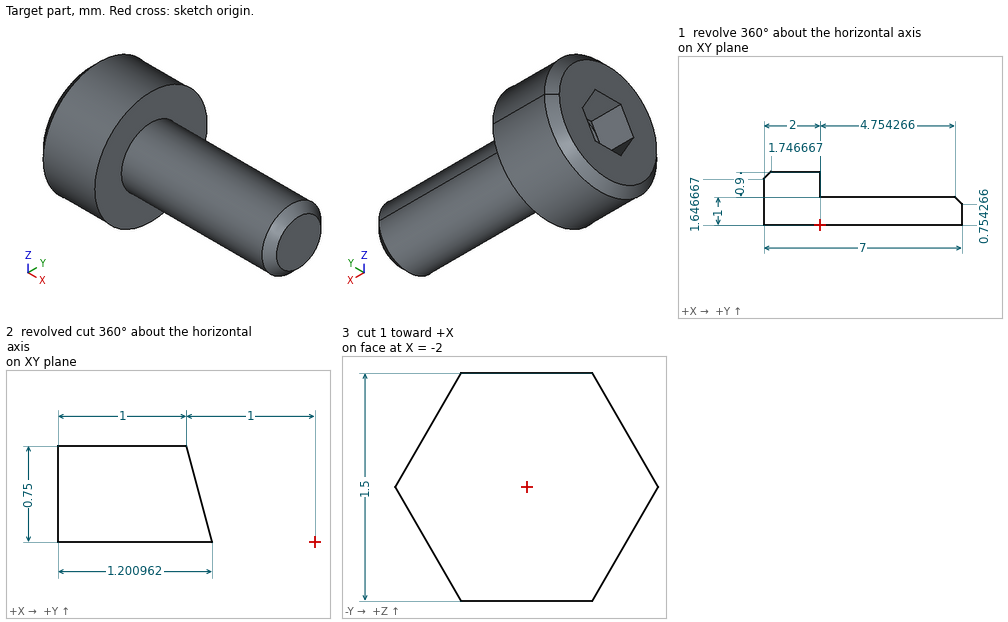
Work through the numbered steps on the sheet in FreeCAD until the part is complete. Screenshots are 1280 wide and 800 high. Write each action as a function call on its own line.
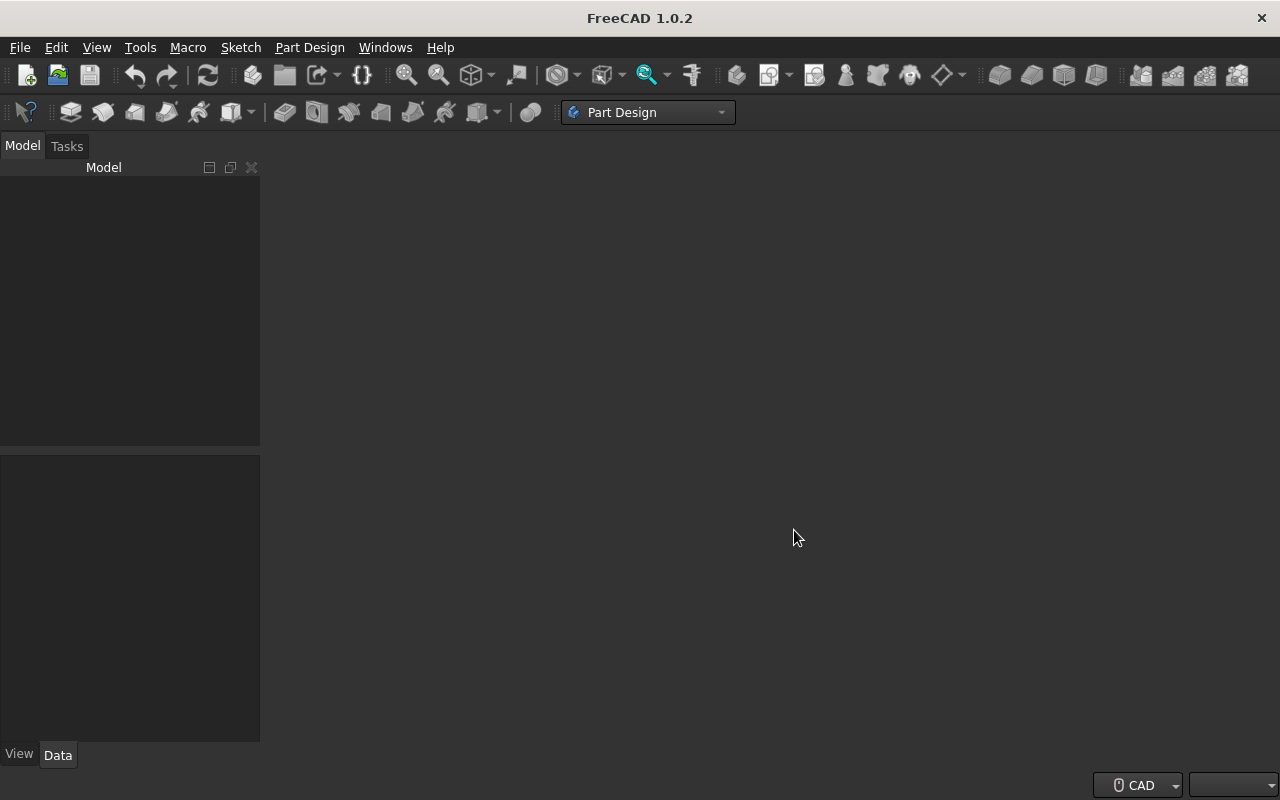
click(26, 76)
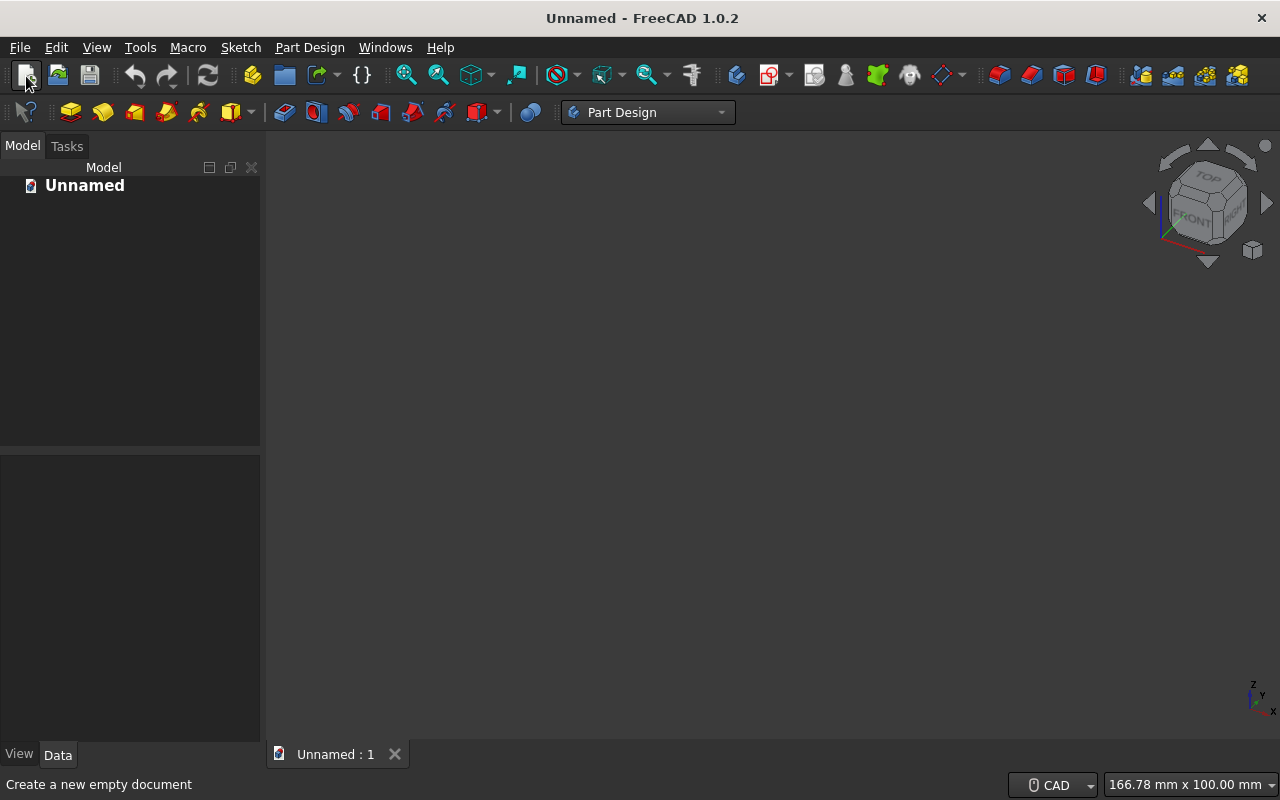
click(770, 76)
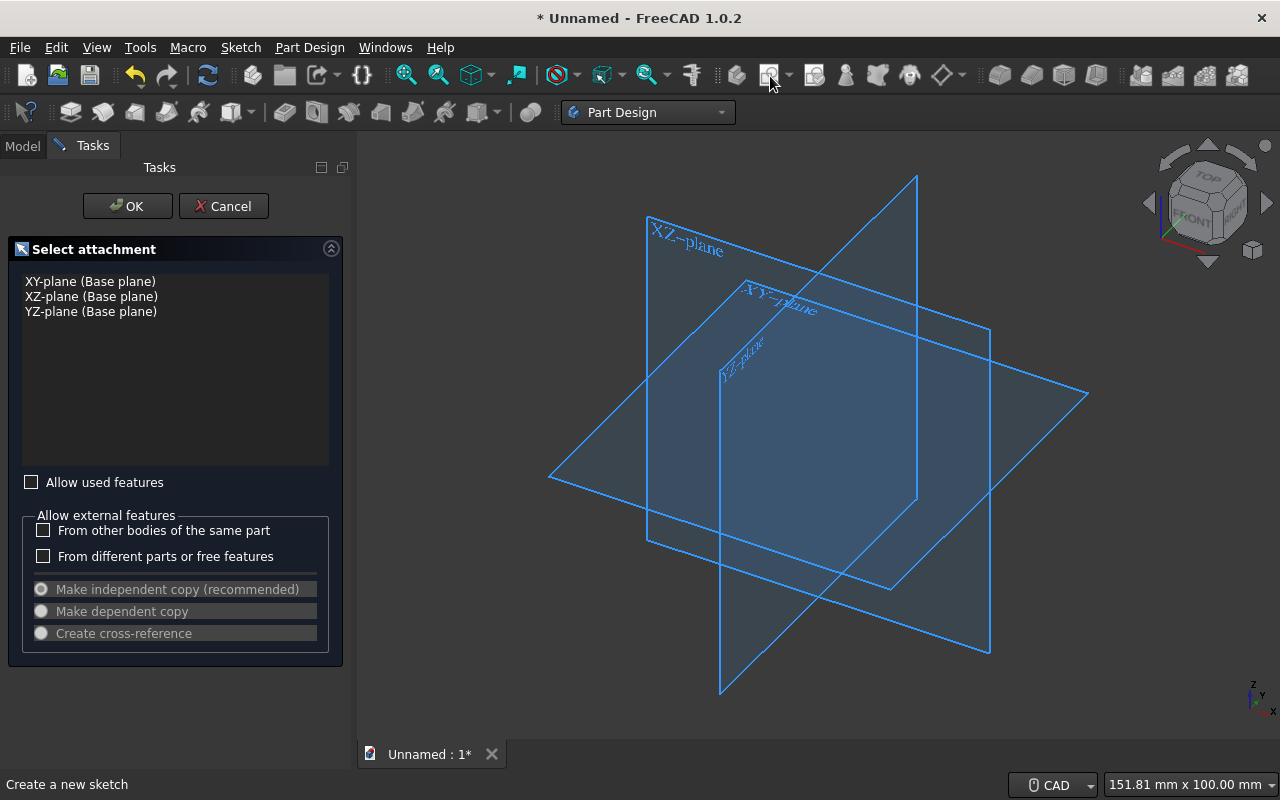
click(82, 282)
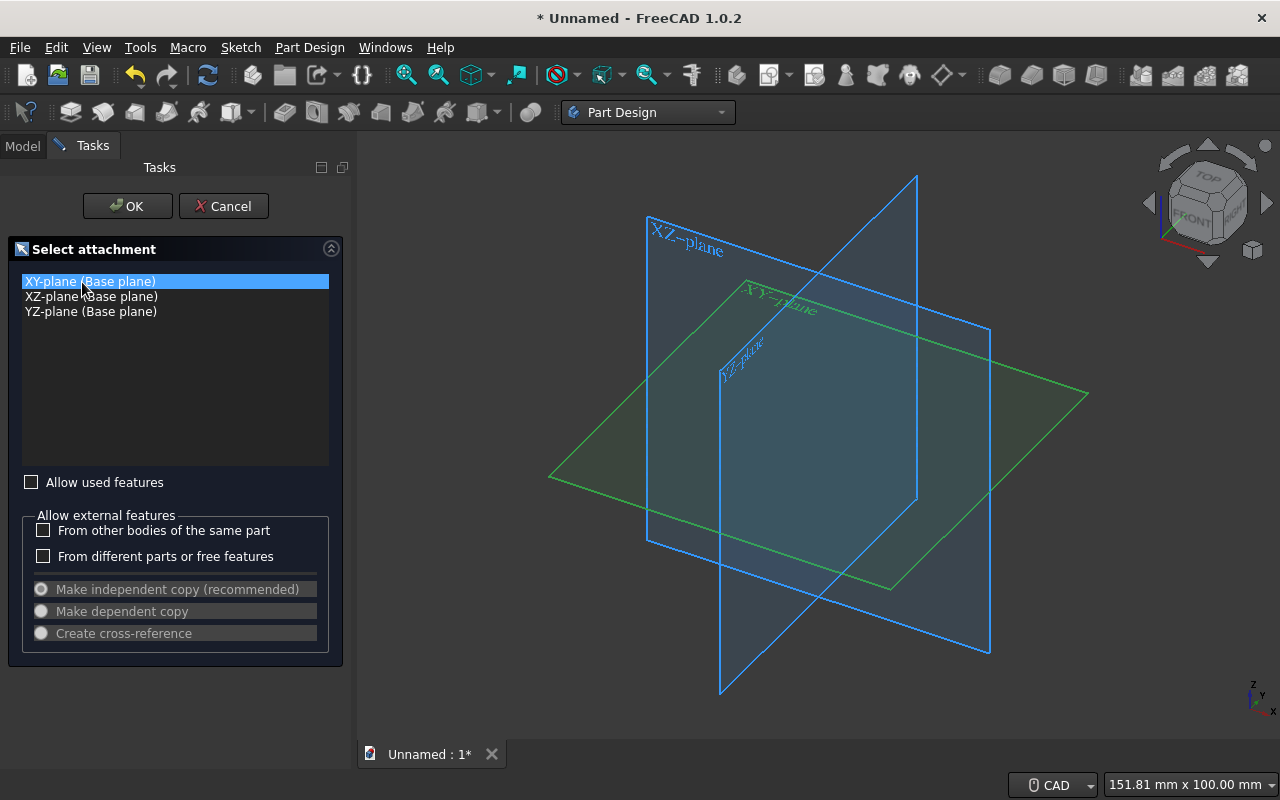
click(128, 206)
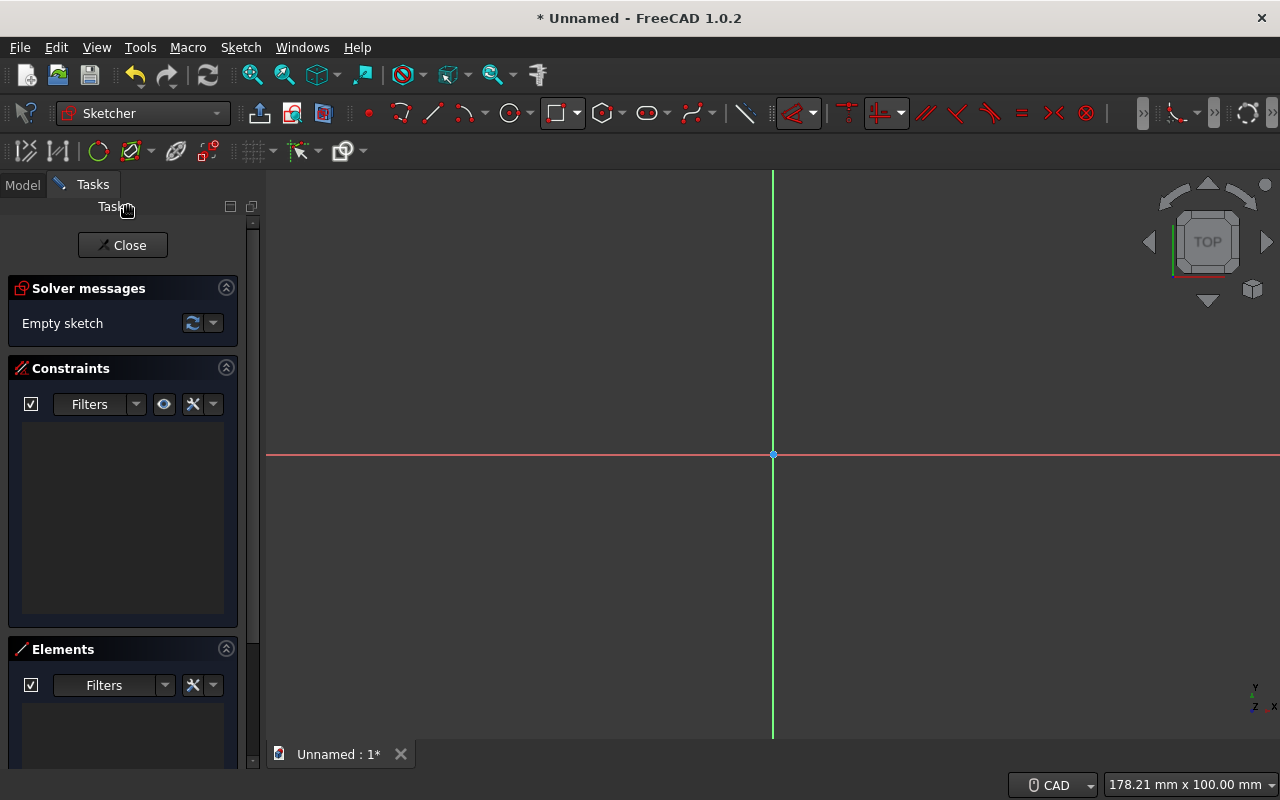
scroll(788, 449, up, 13)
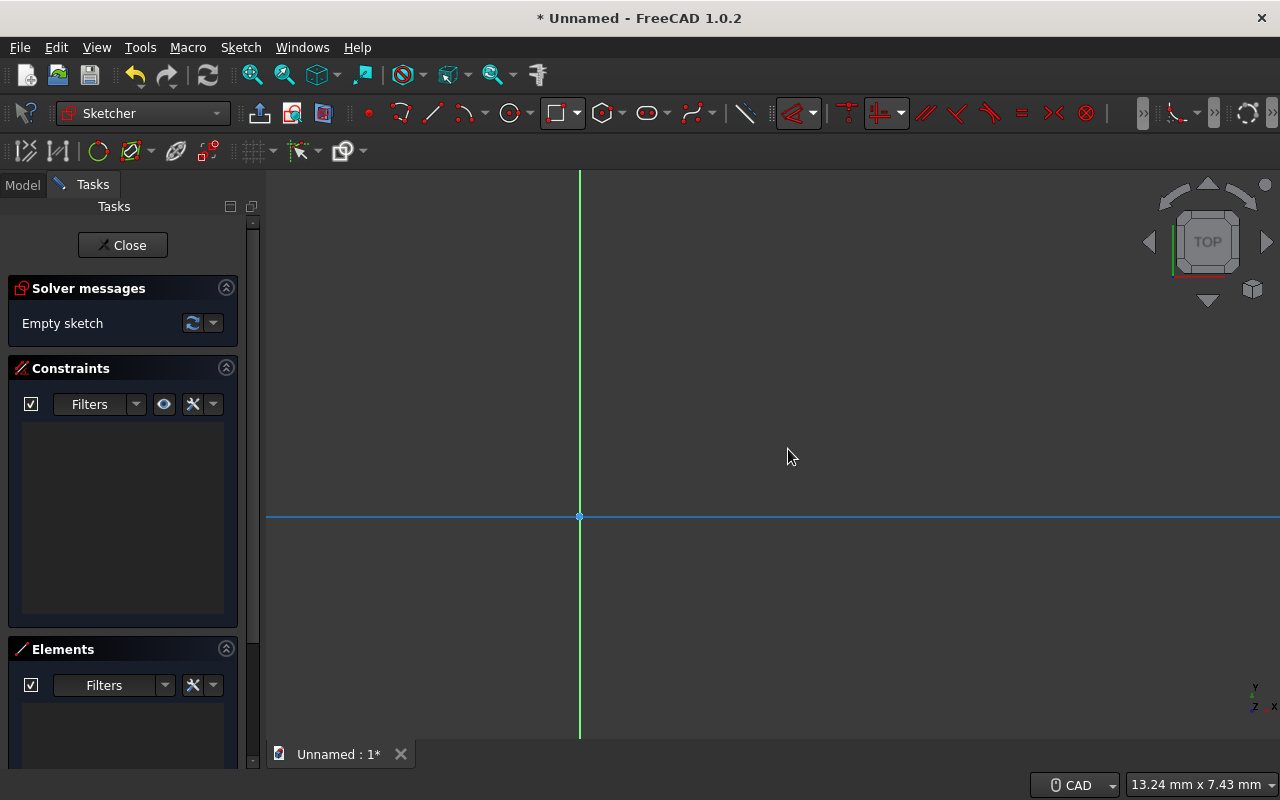
click(402, 114)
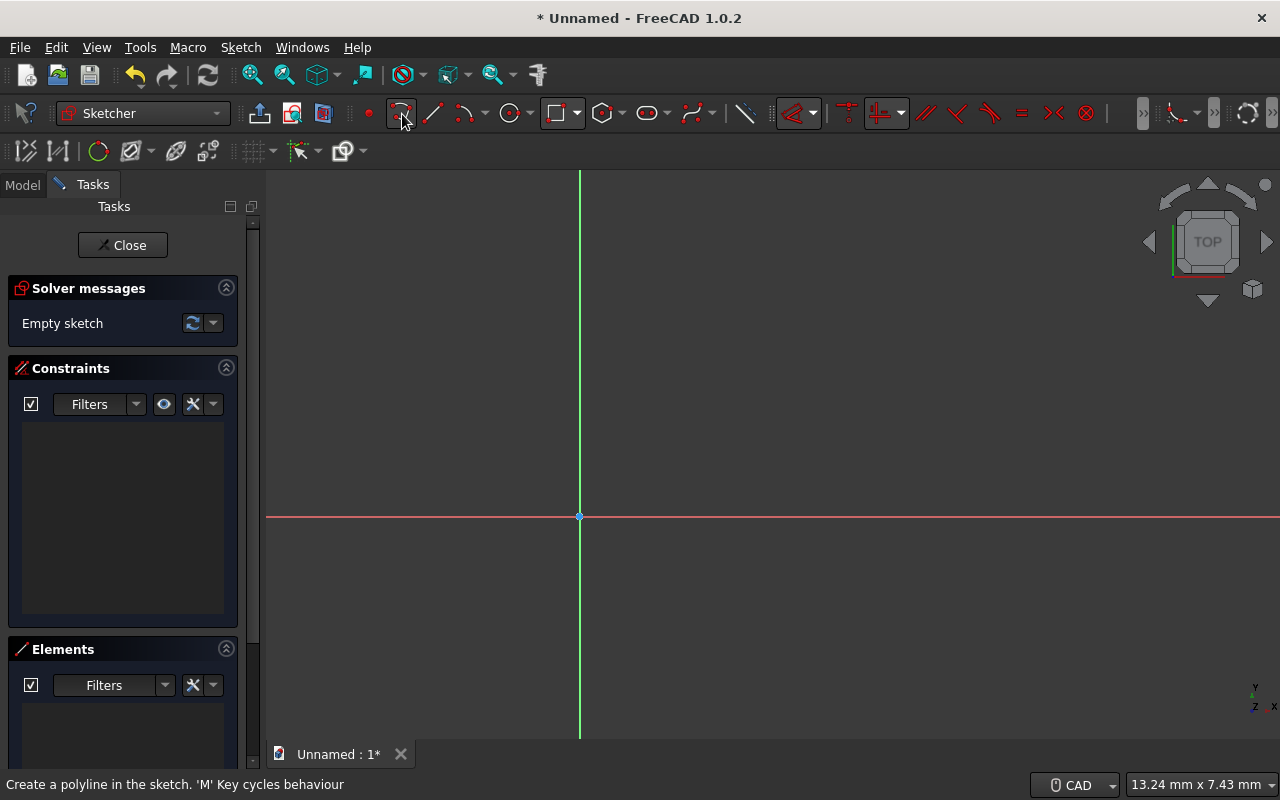
click(580, 440)
click(589, 371)
click(446, 371)
click(426, 391)
click(426, 517)
click(963, 508)
click(963, 459)
click(944, 440)
click(580, 441)
key(Escape)
key(Escape)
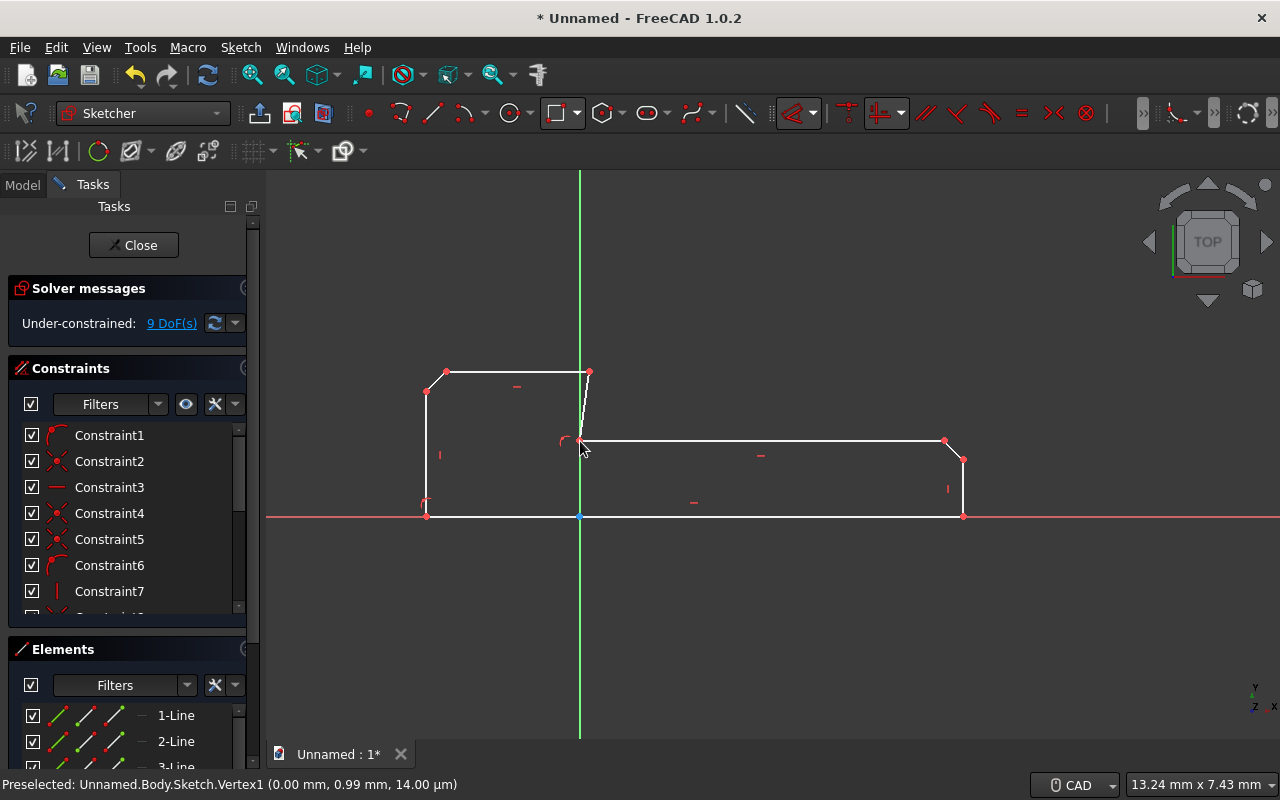
click(582, 420)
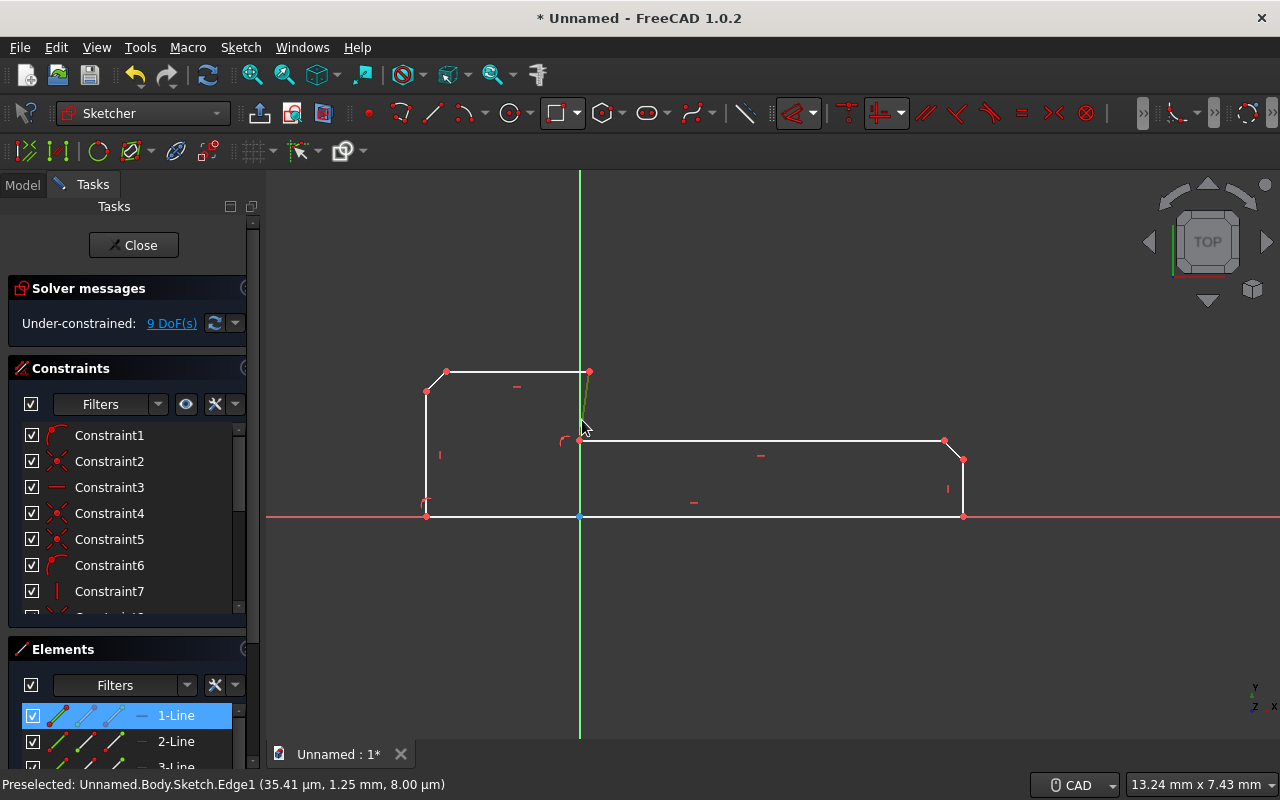
key(v)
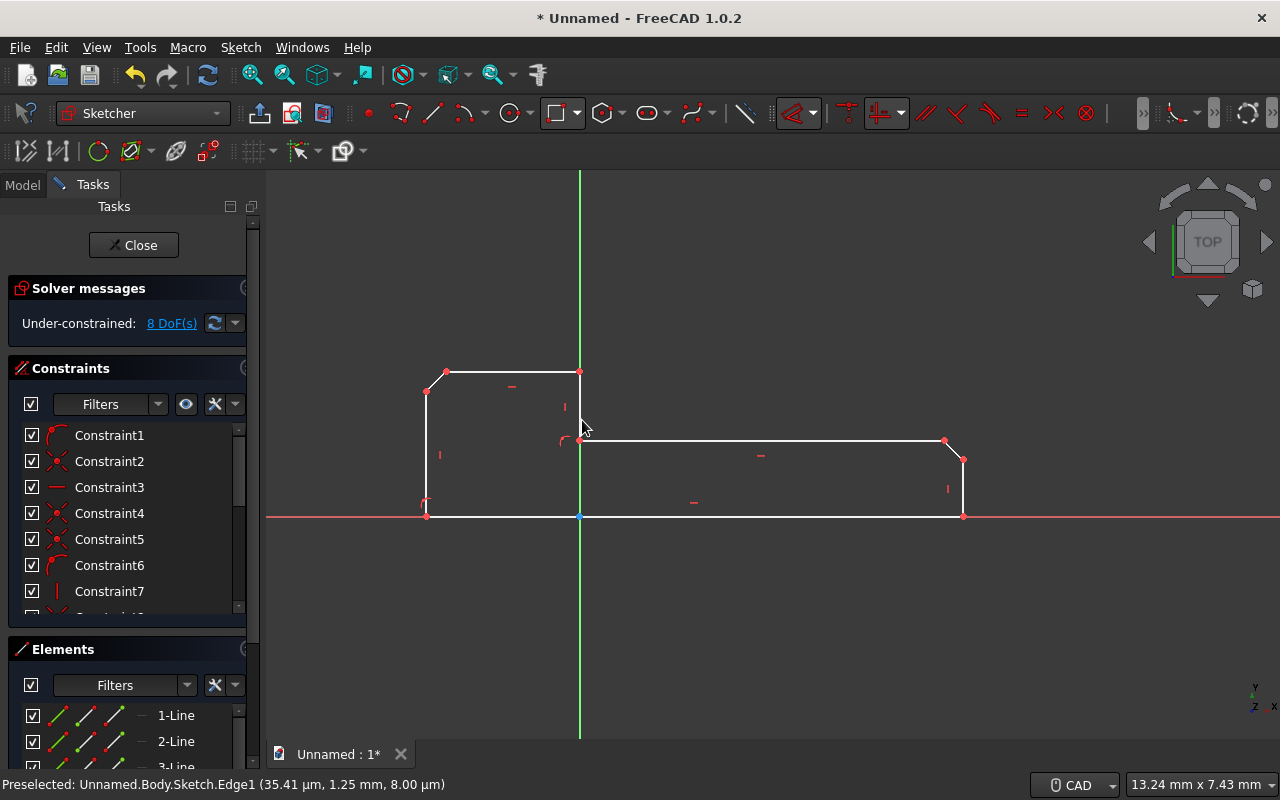
click(792, 114)